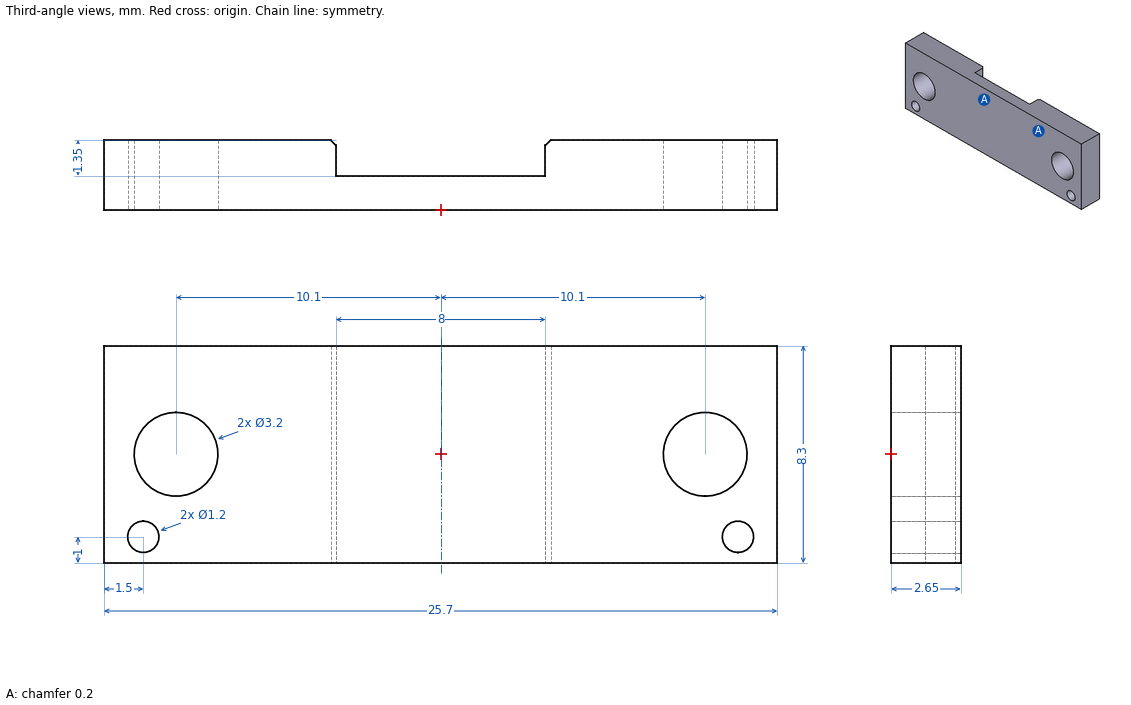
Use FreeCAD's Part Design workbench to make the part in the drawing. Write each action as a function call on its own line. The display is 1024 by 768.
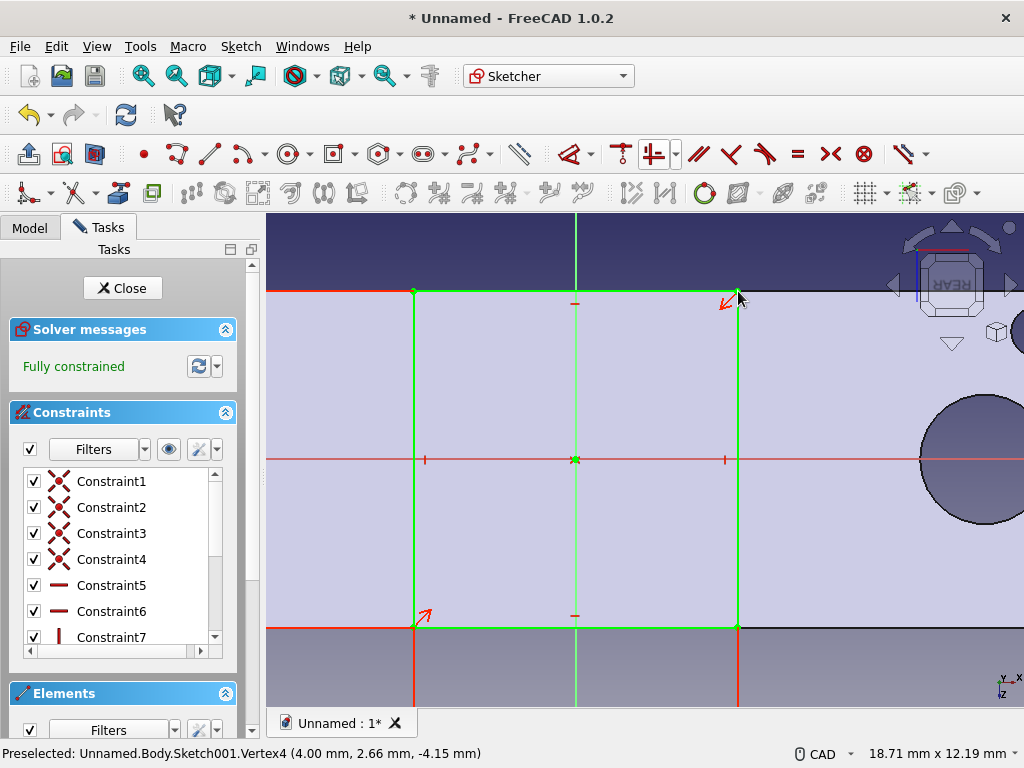
click(123, 288)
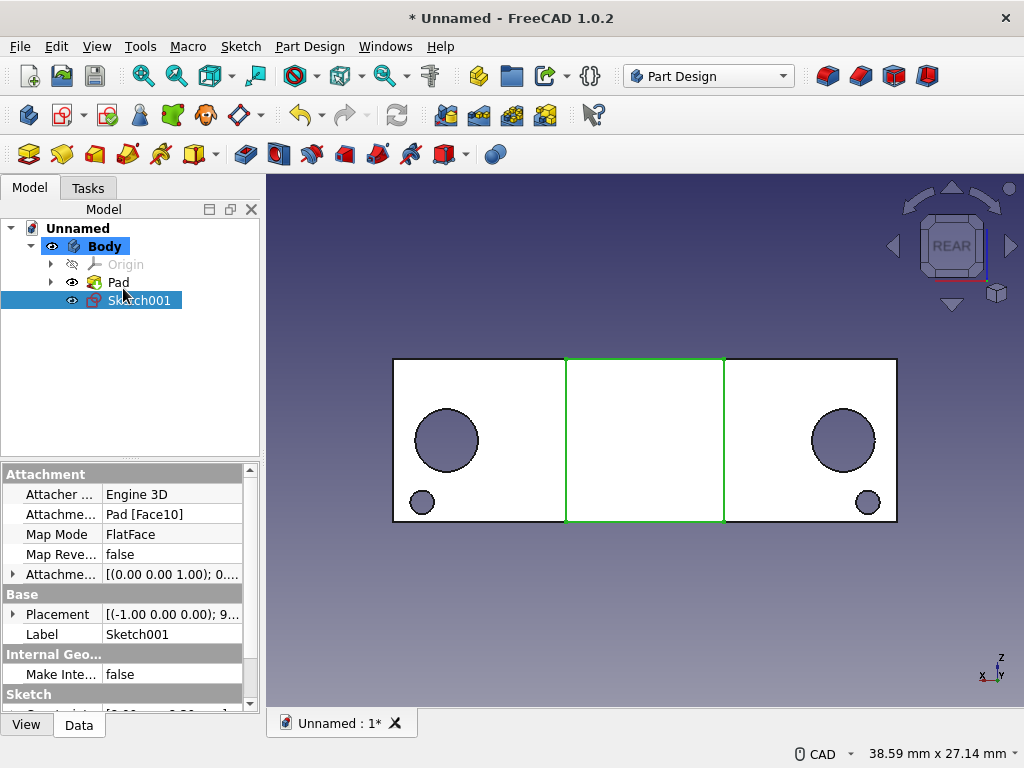
click(246, 154)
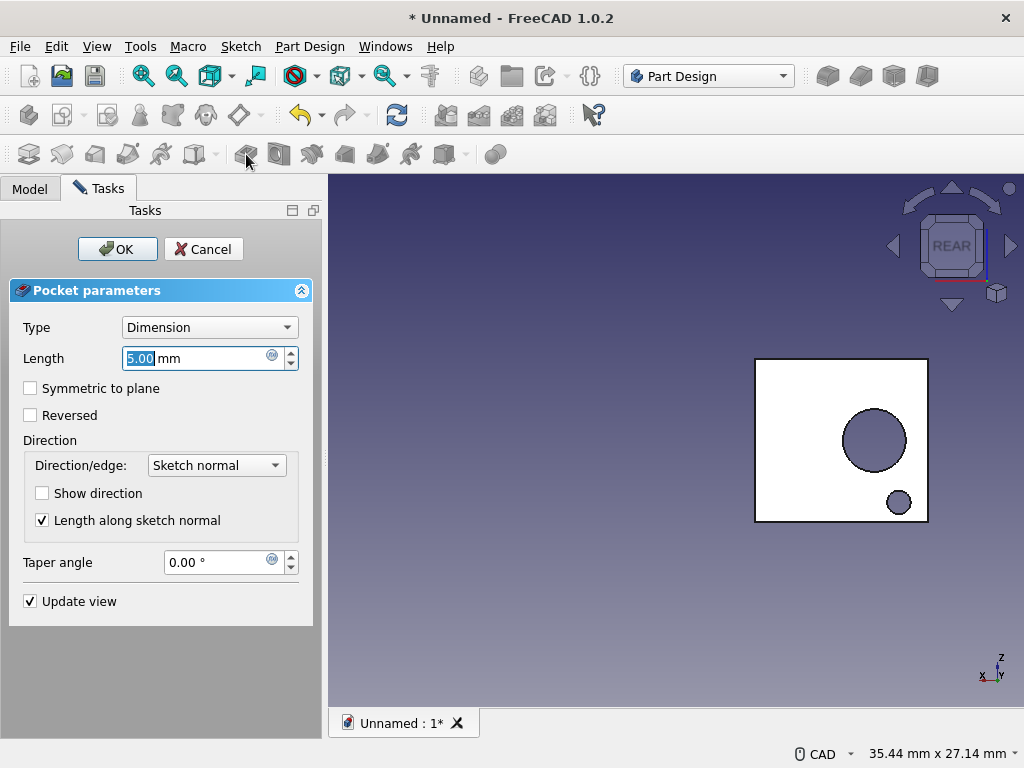
text(1.35)
key(Tab)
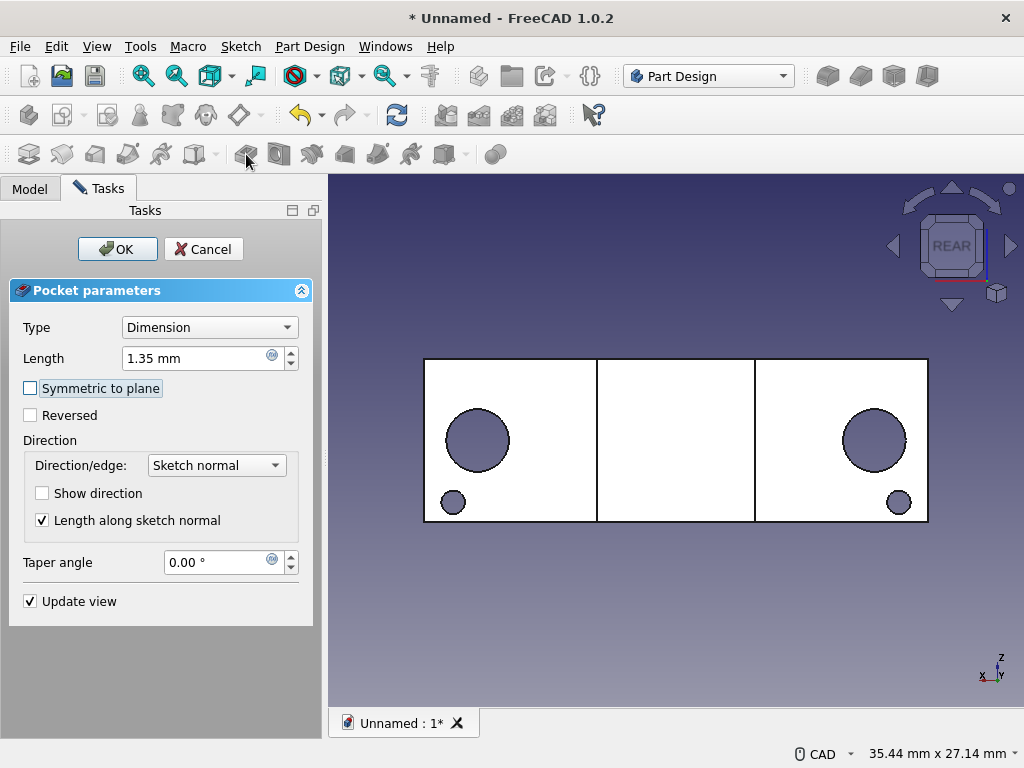
click(118, 249)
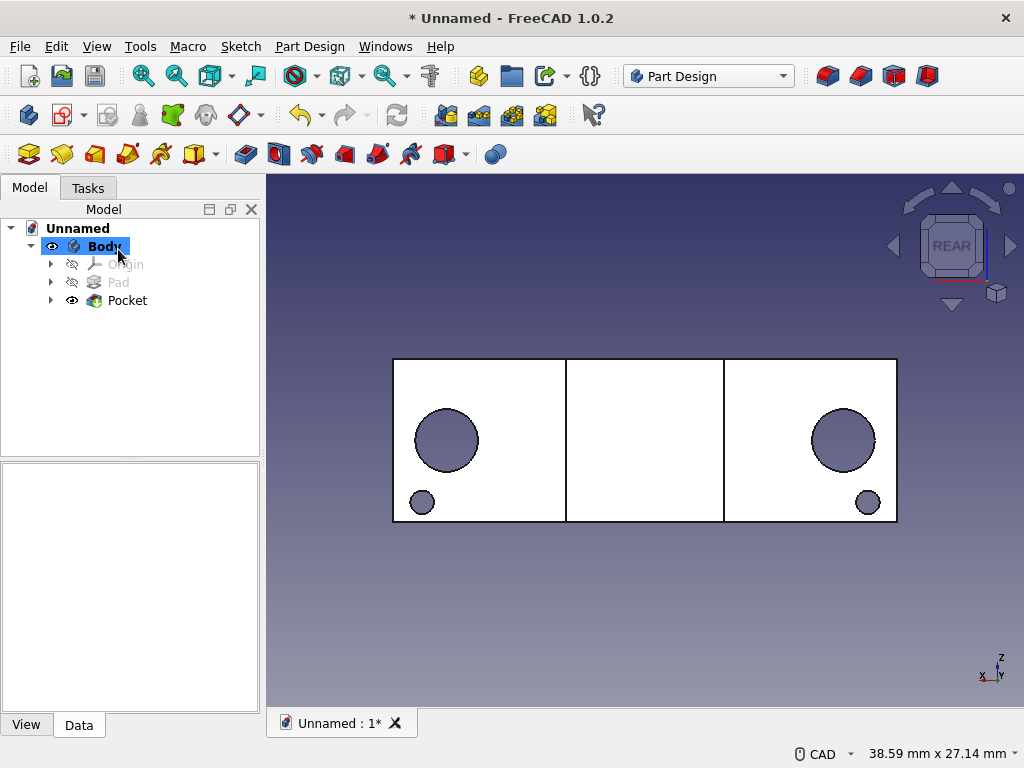
click(566, 439)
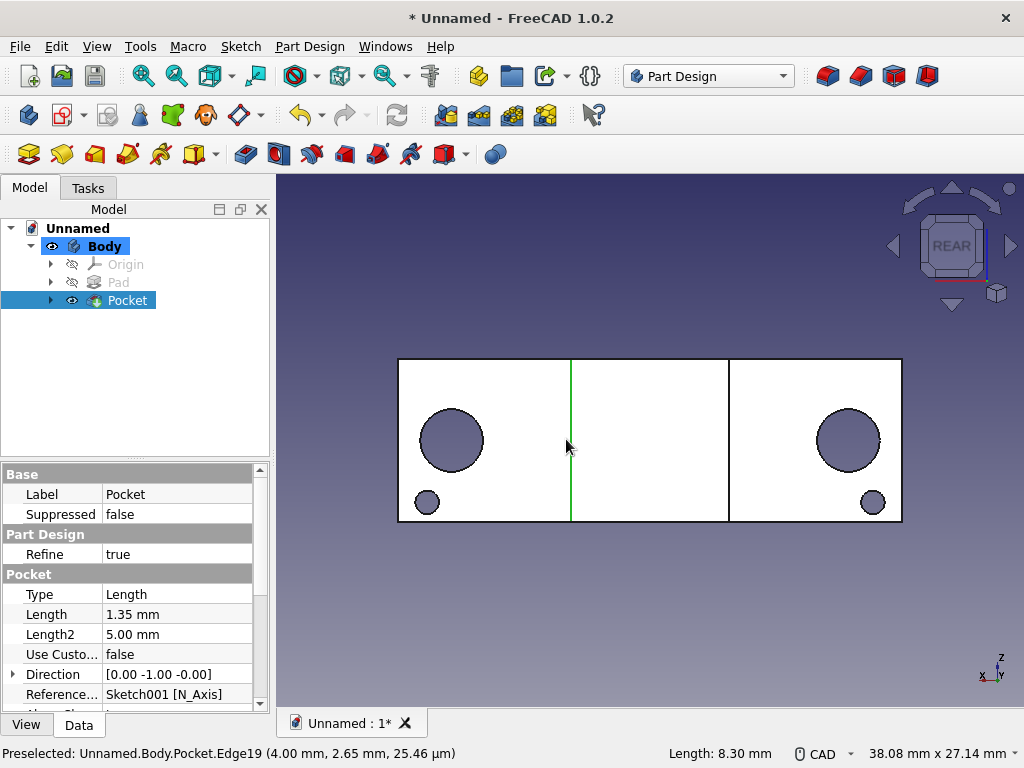
key(0)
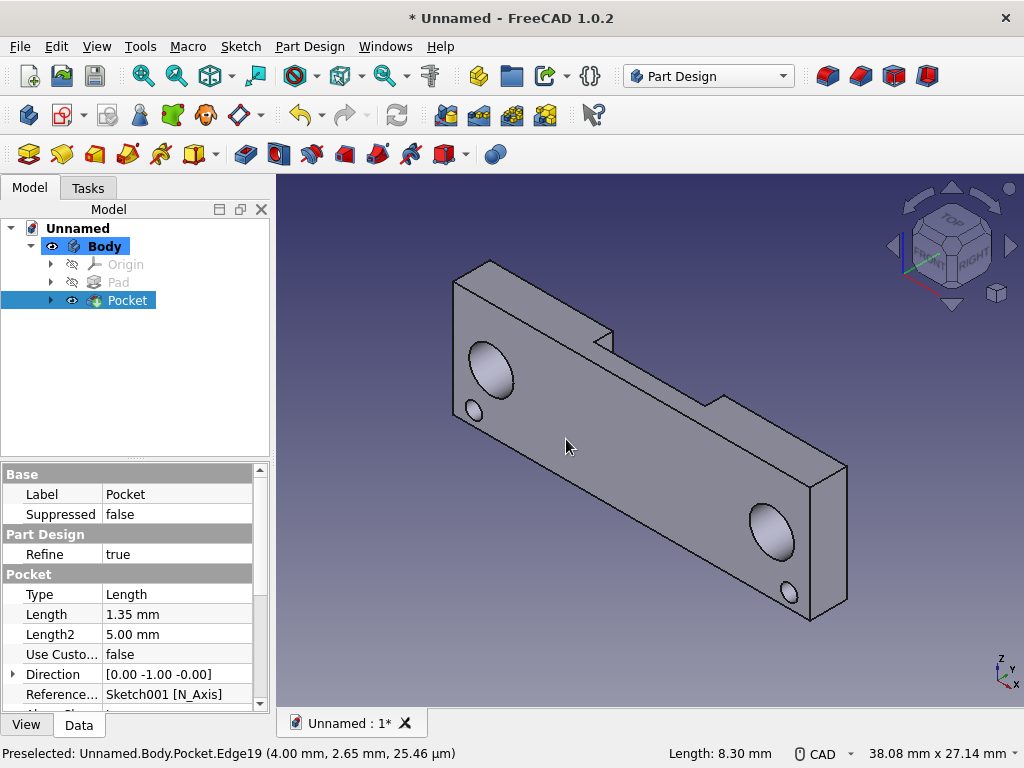
key(2)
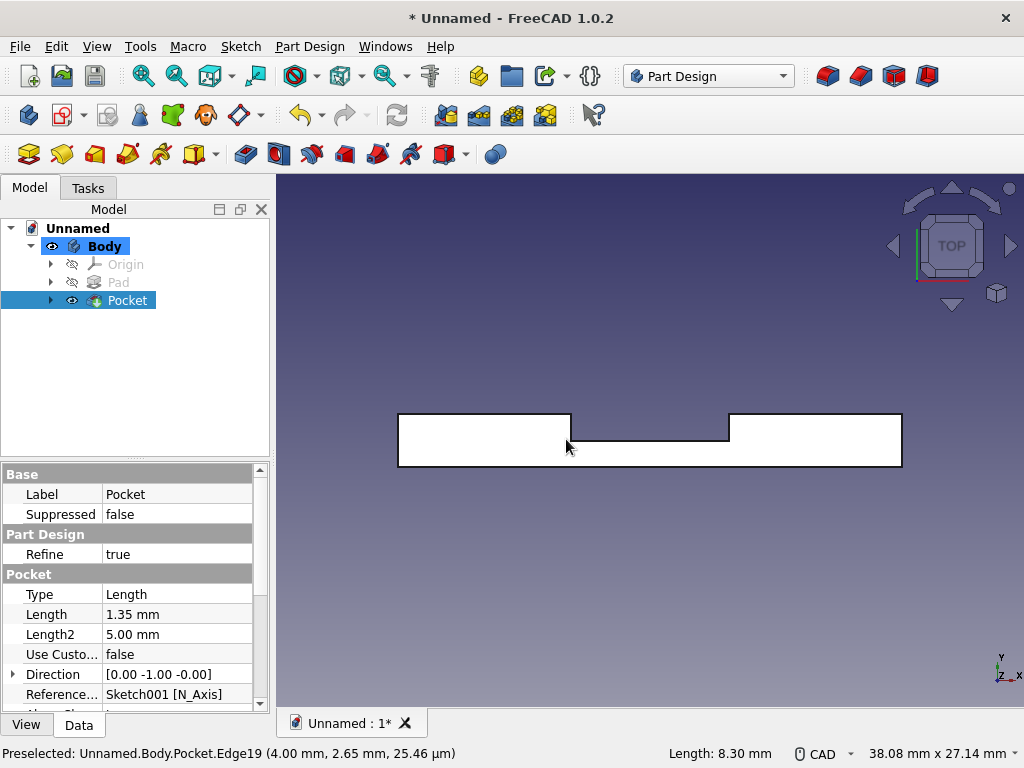
key(1)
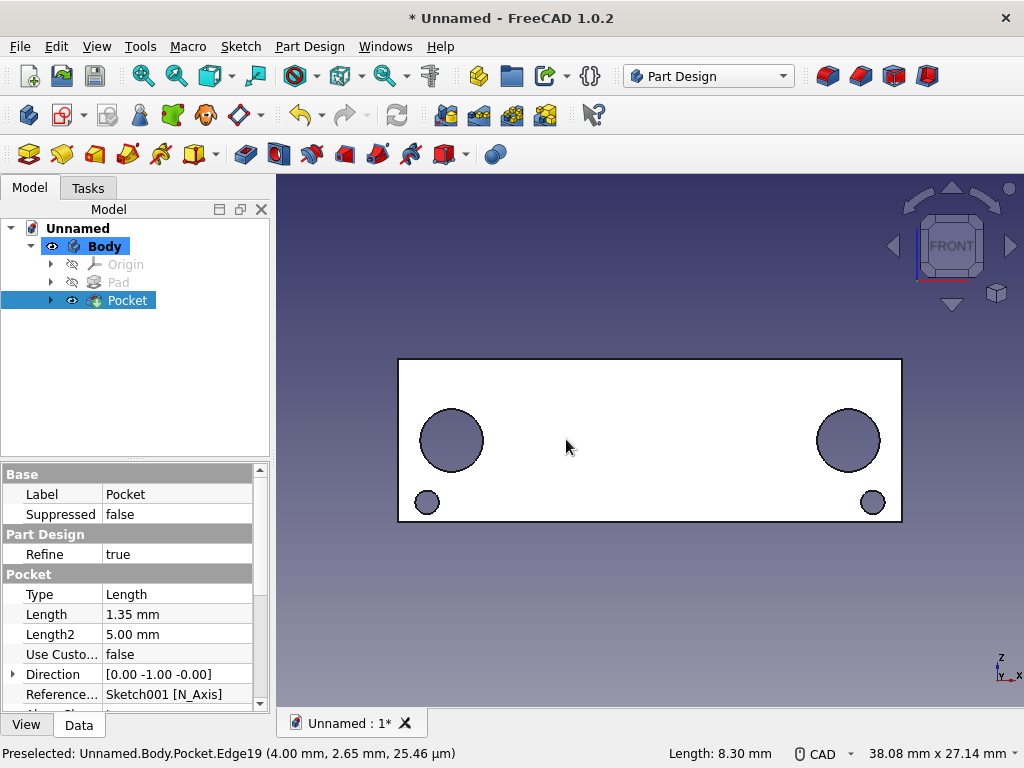
key(3)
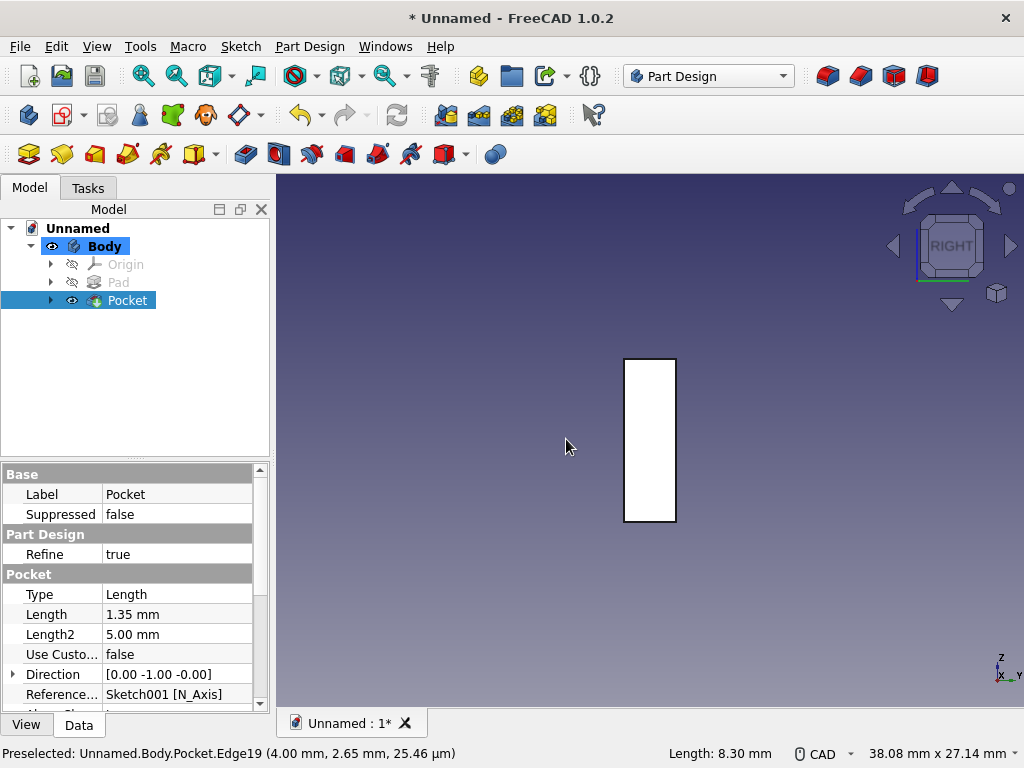
click(144, 76)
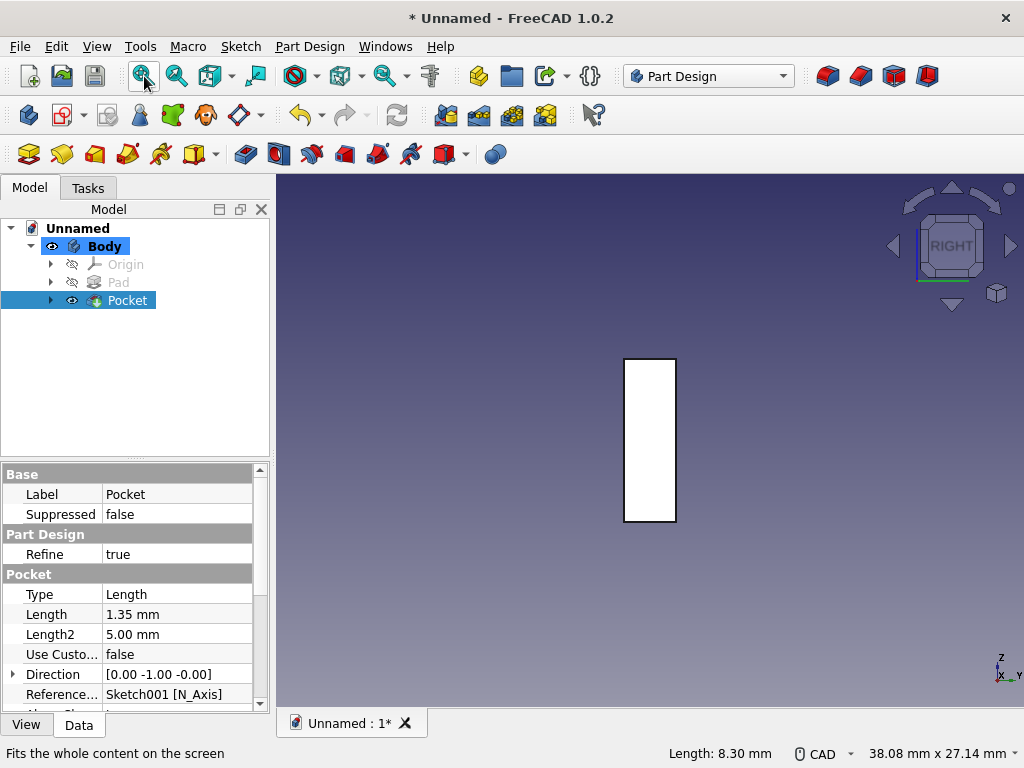
key(5)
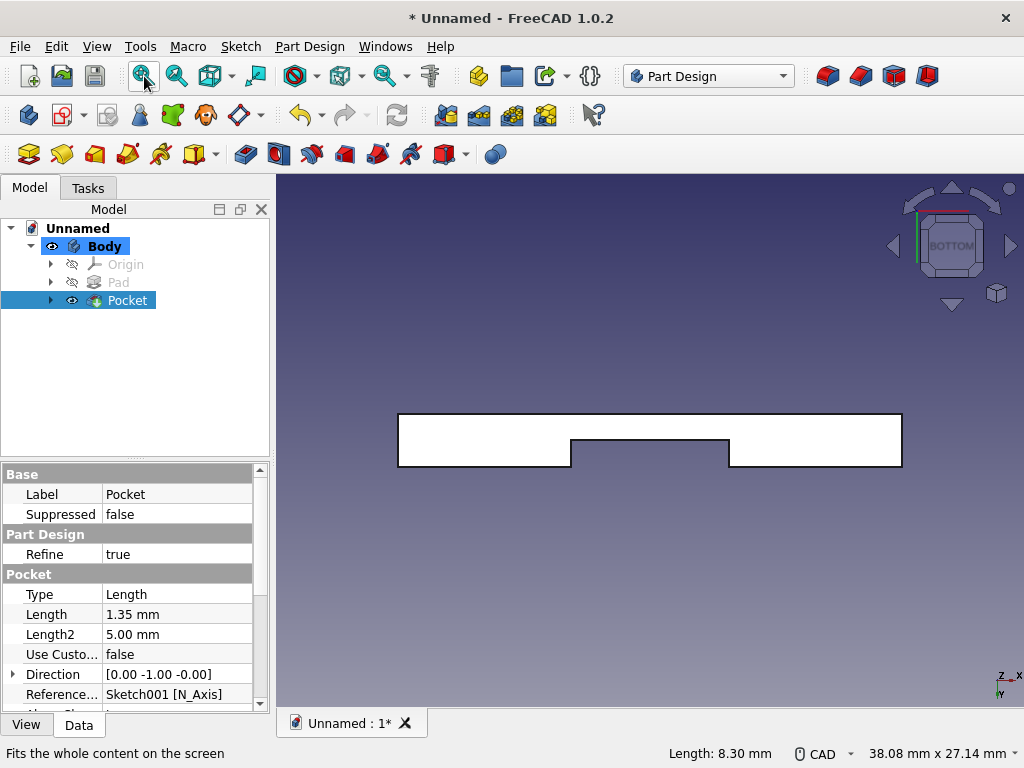
key(4)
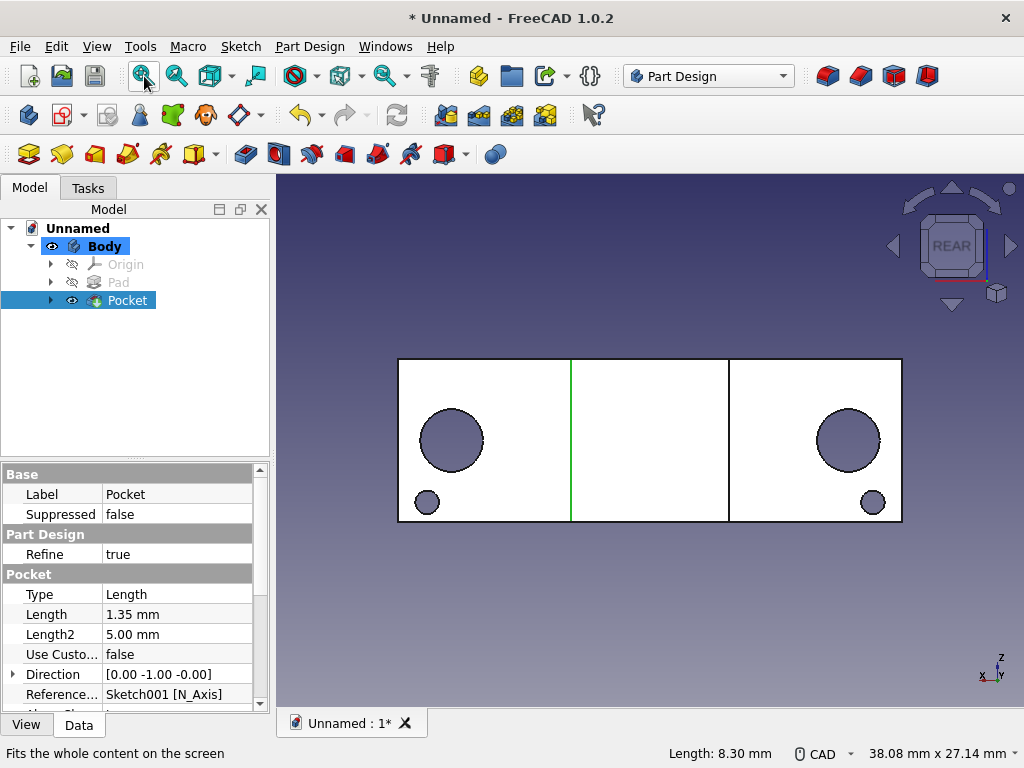
click(729, 439, ctrl)